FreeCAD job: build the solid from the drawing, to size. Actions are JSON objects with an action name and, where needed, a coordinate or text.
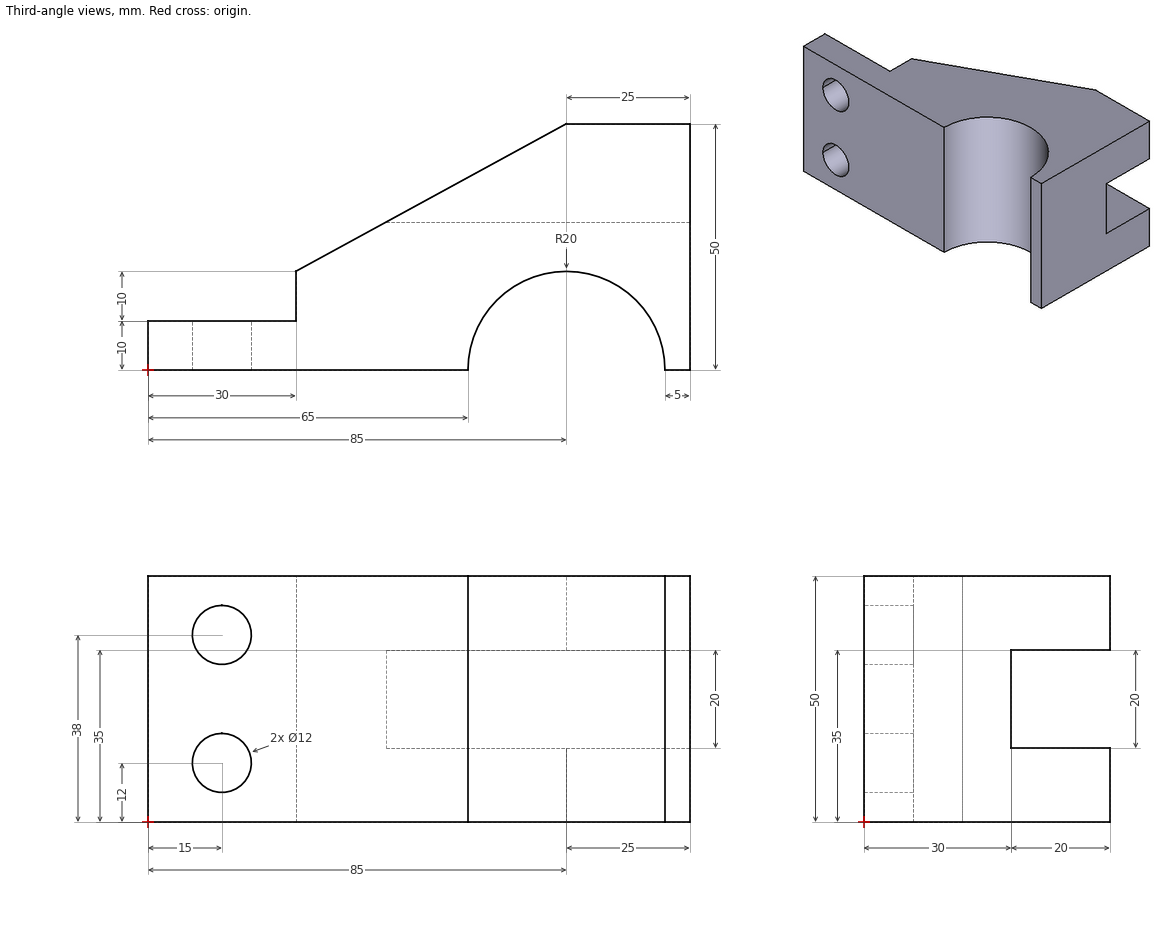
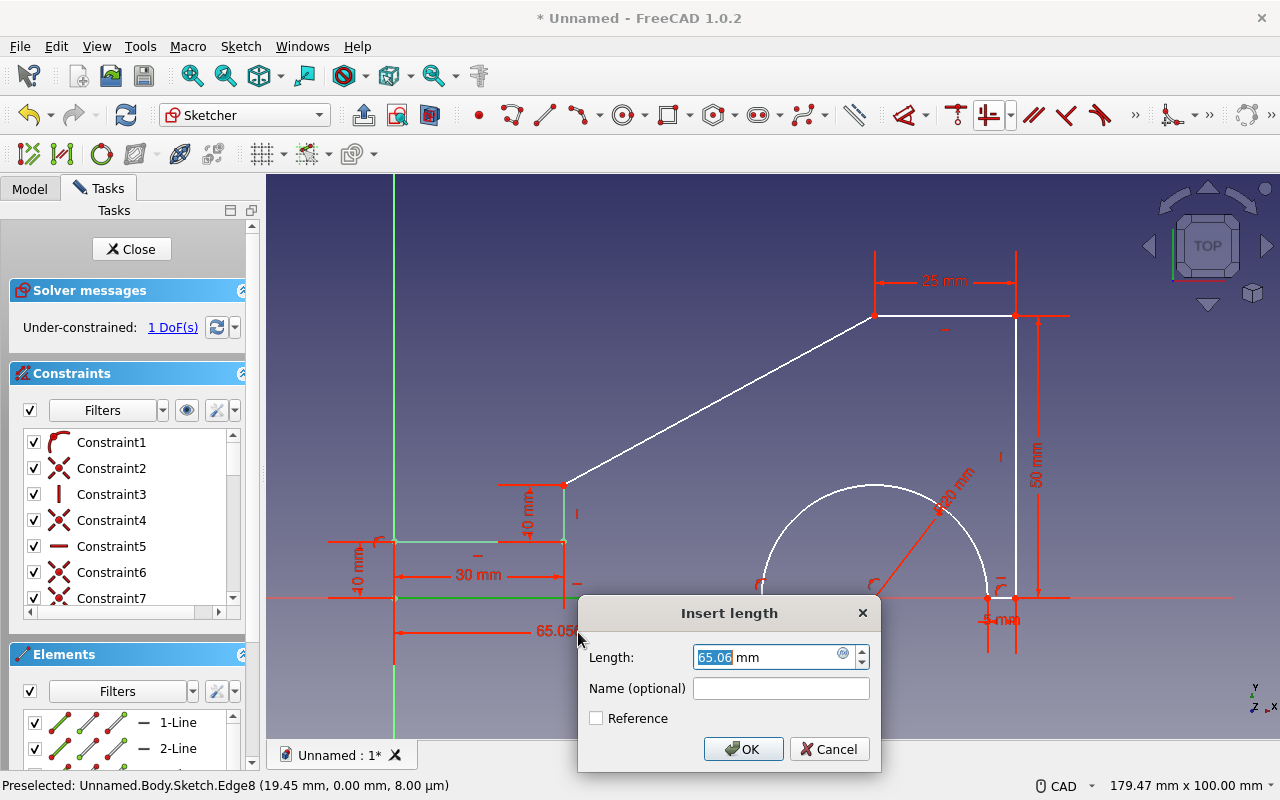
{"action": "type", "text": "65"}
{"action": "key", "text": "Return"}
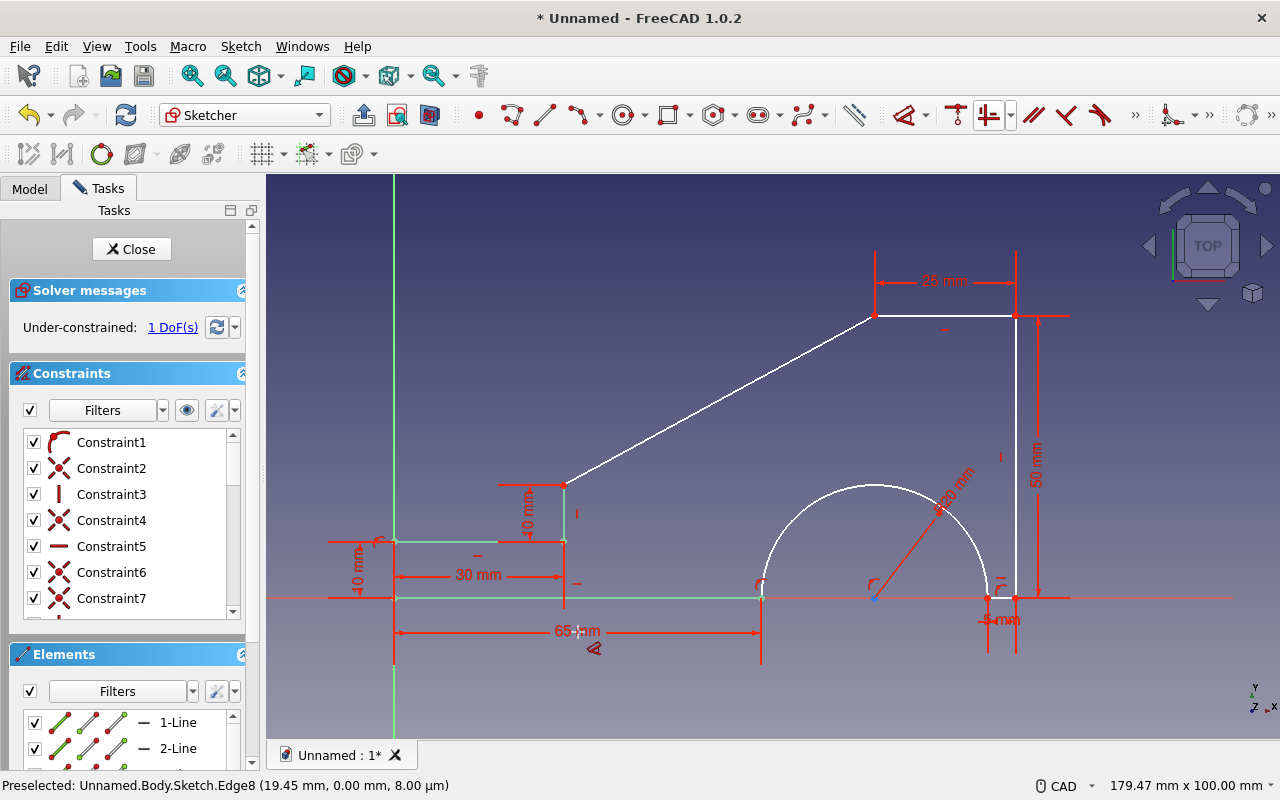
{"action": "left_click", "coordinate": [875, 316]}
{"action": "left_click", "coordinate": [745, 632]}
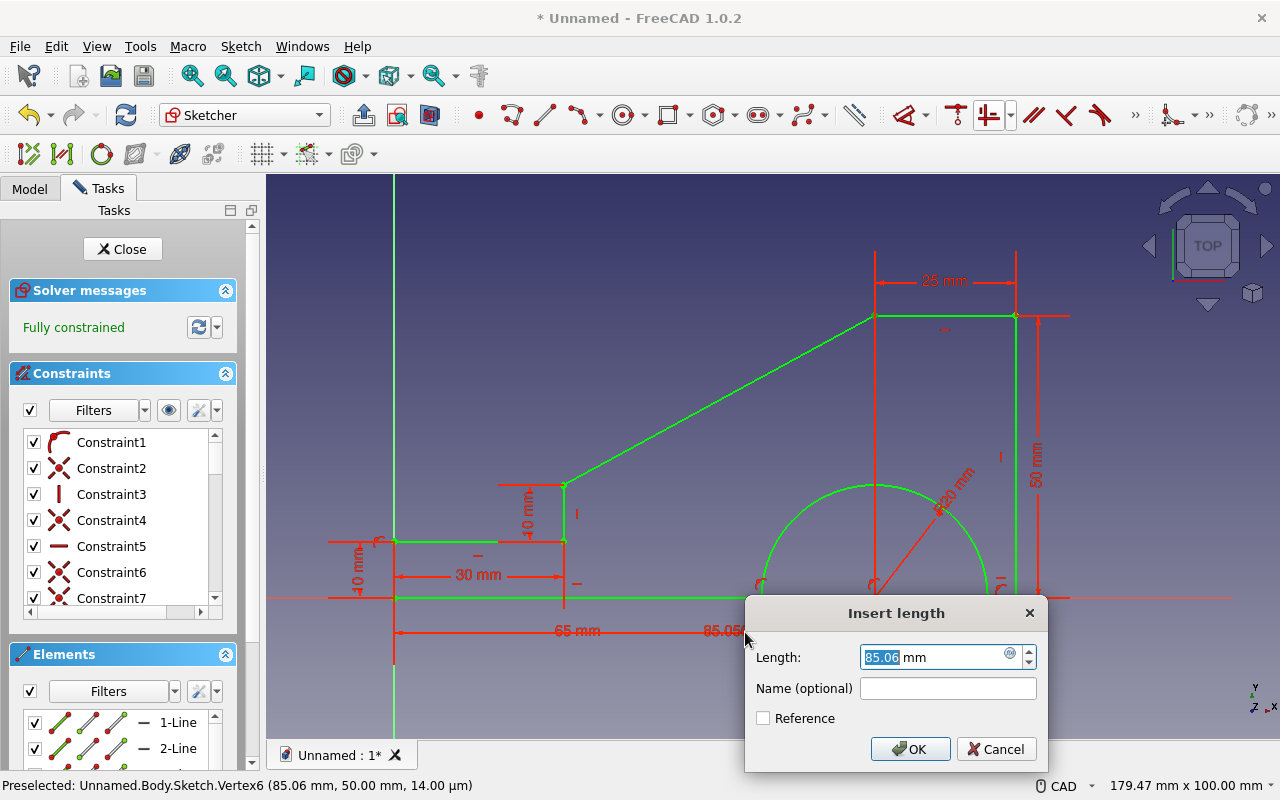
{"action": "type", "text": "85"}
{"action": "key", "text": "Return"}
{"action": "key", "text": "Escape"}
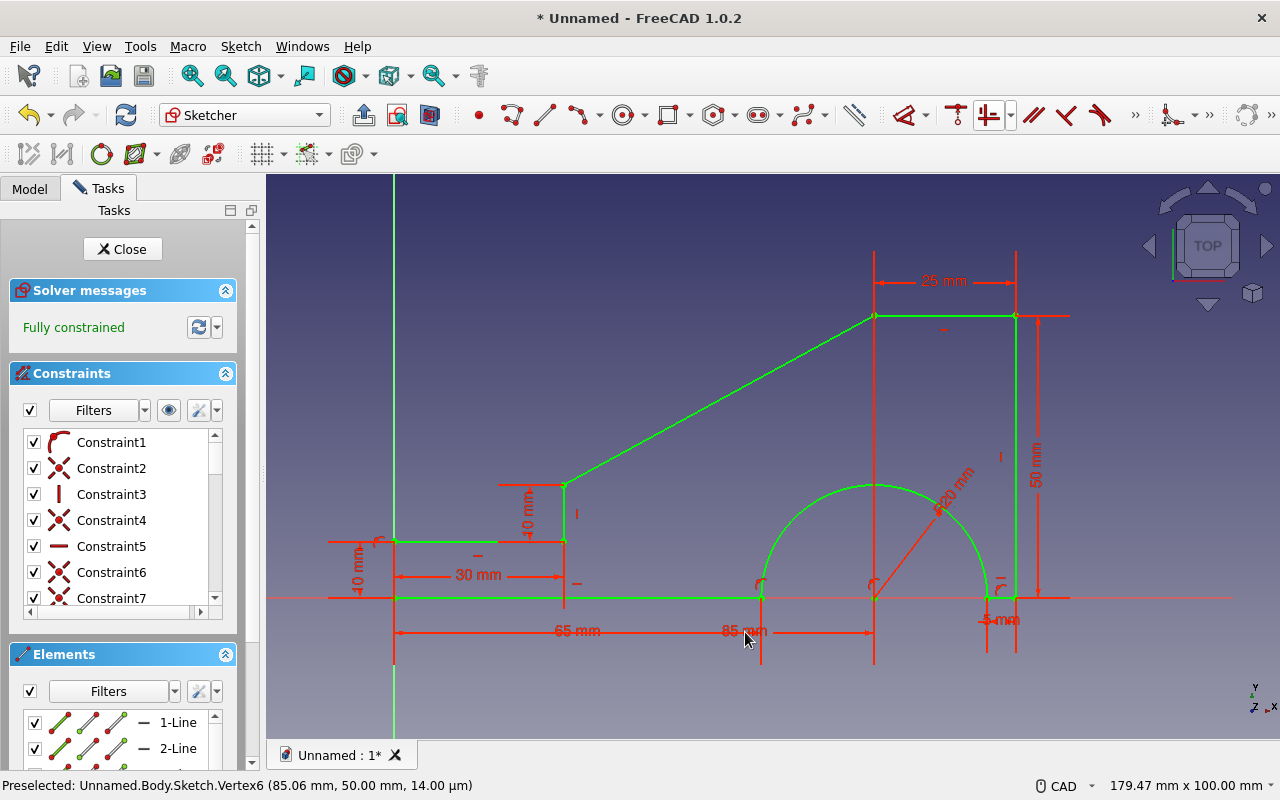
{"action": "left_click", "coordinate": [123, 249]}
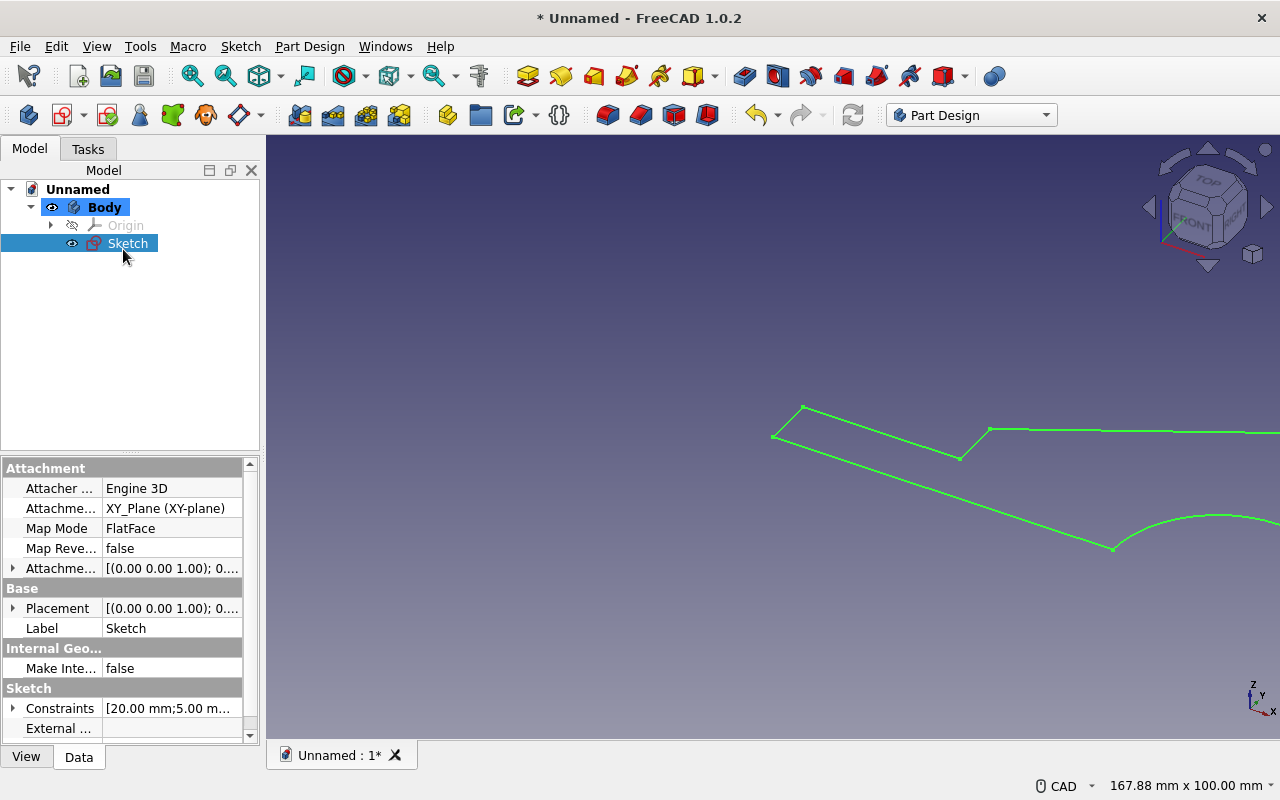
{"action": "left_click", "coordinate": [528, 76]}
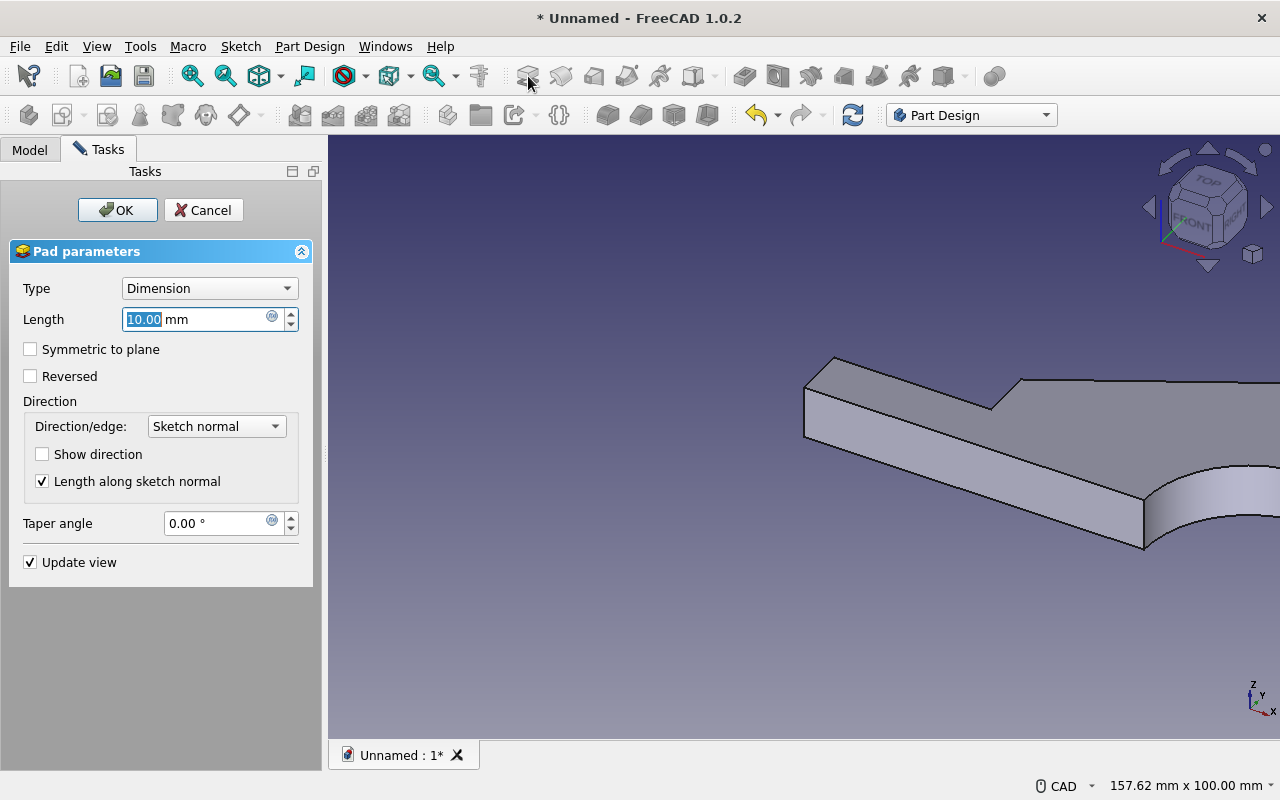
{"action": "type", "text": "50"}
{"action": "key", "text": "Tab"}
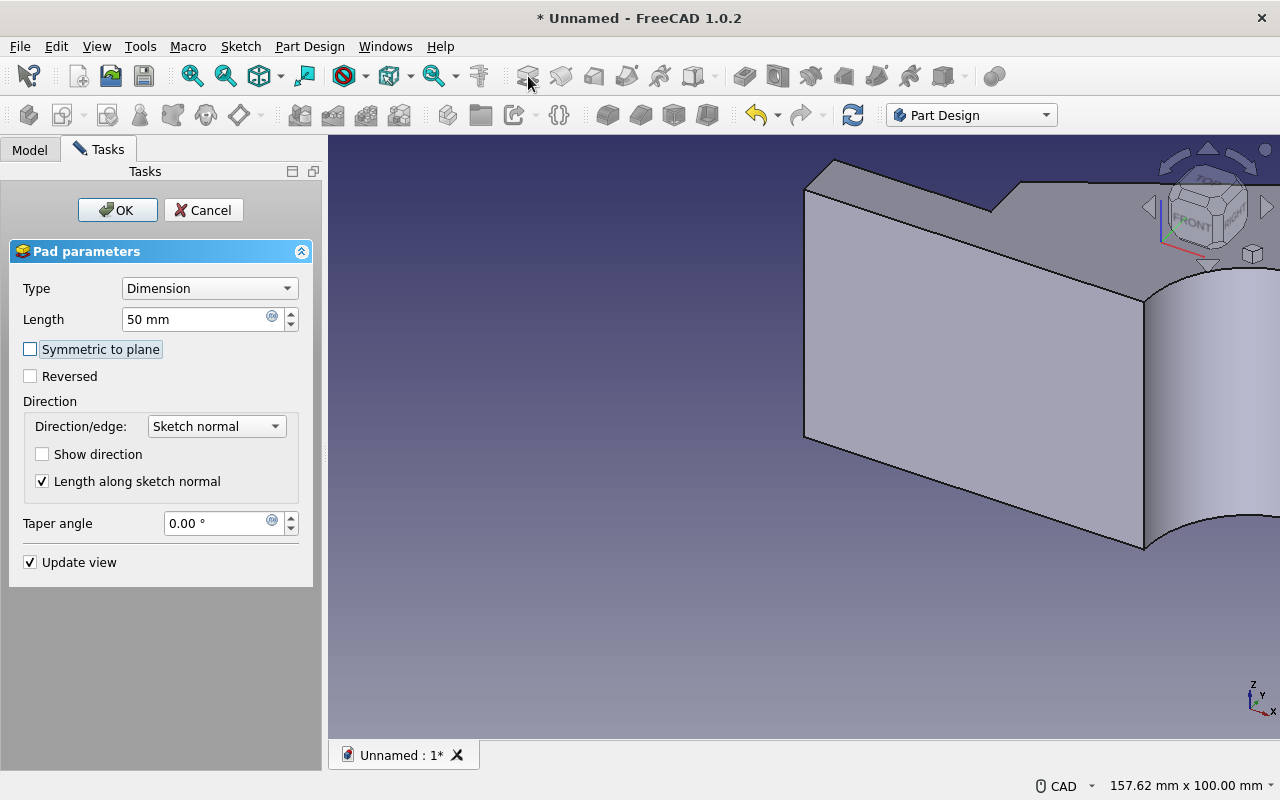
{"action": "left_click", "coordinate": [118, 210]}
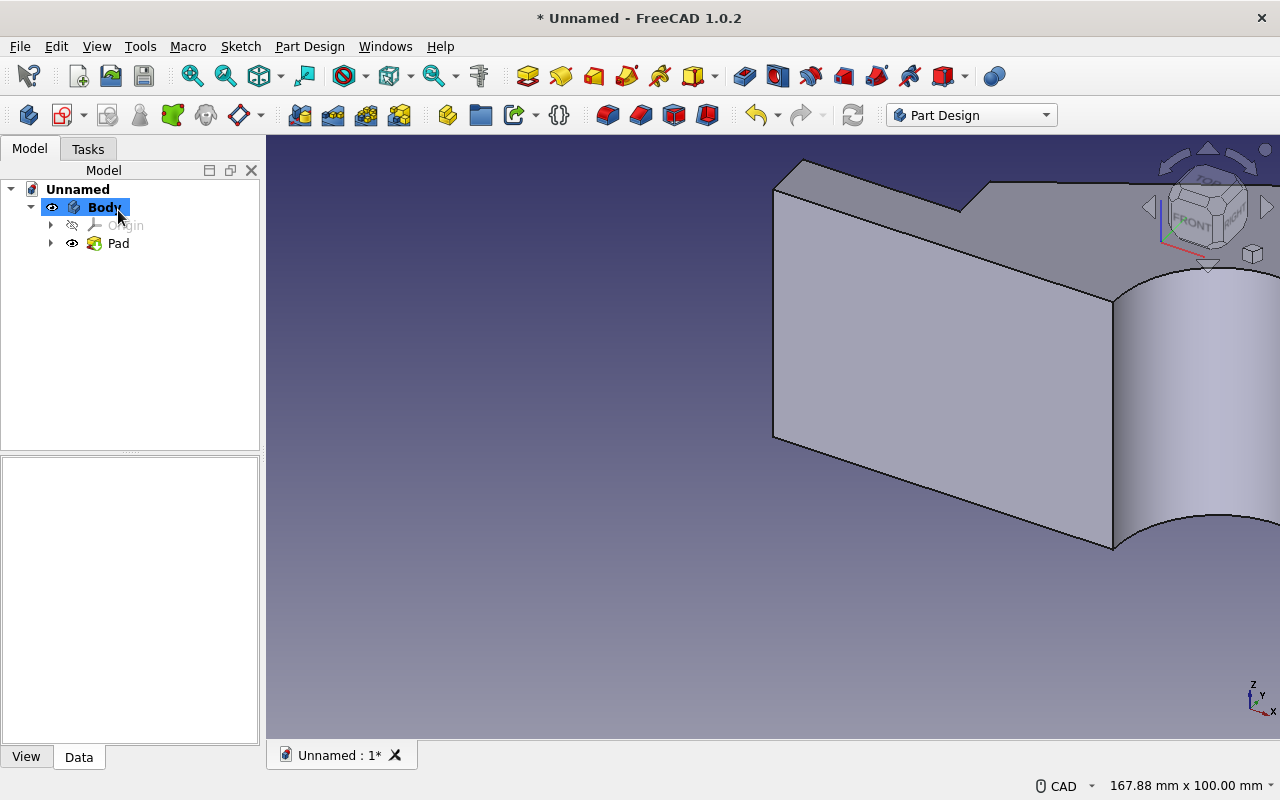
{"action": "left_click", "coordinate": [193, 76]}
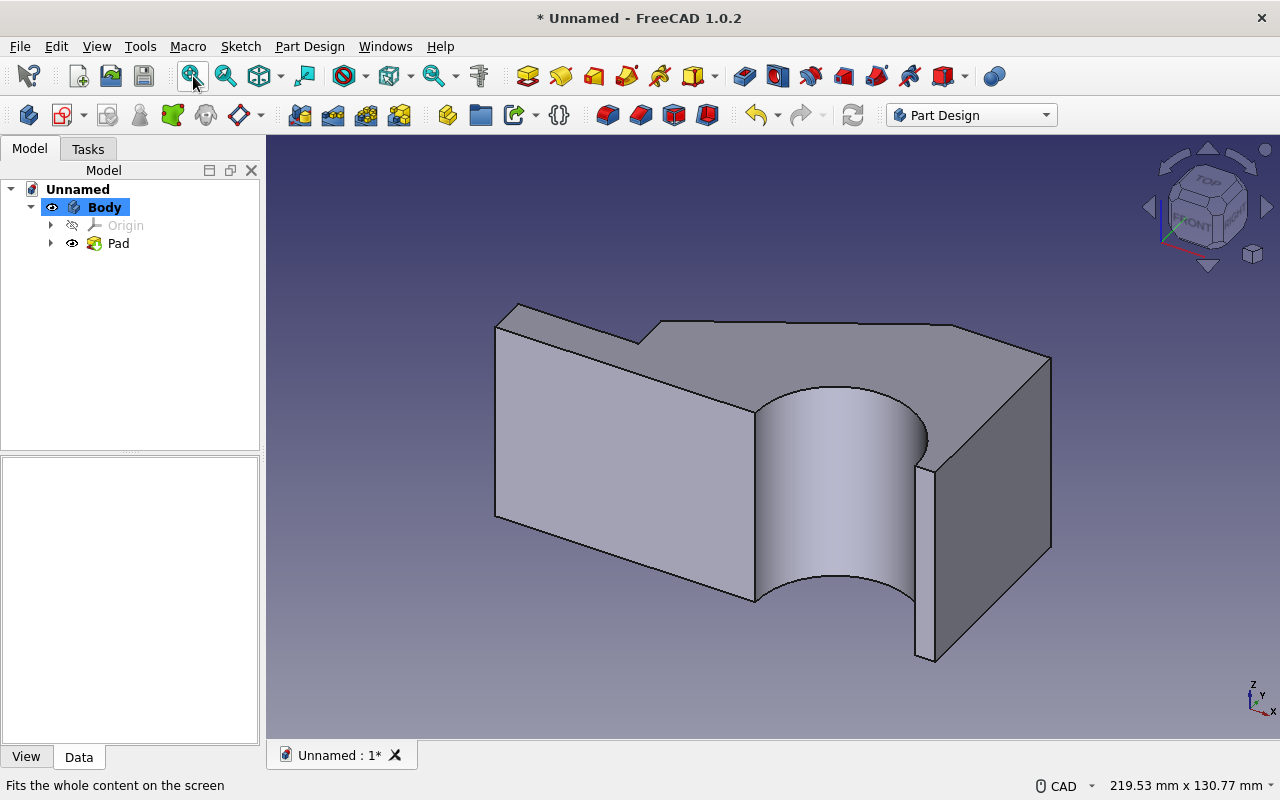
{"action": "key", "text": "4"}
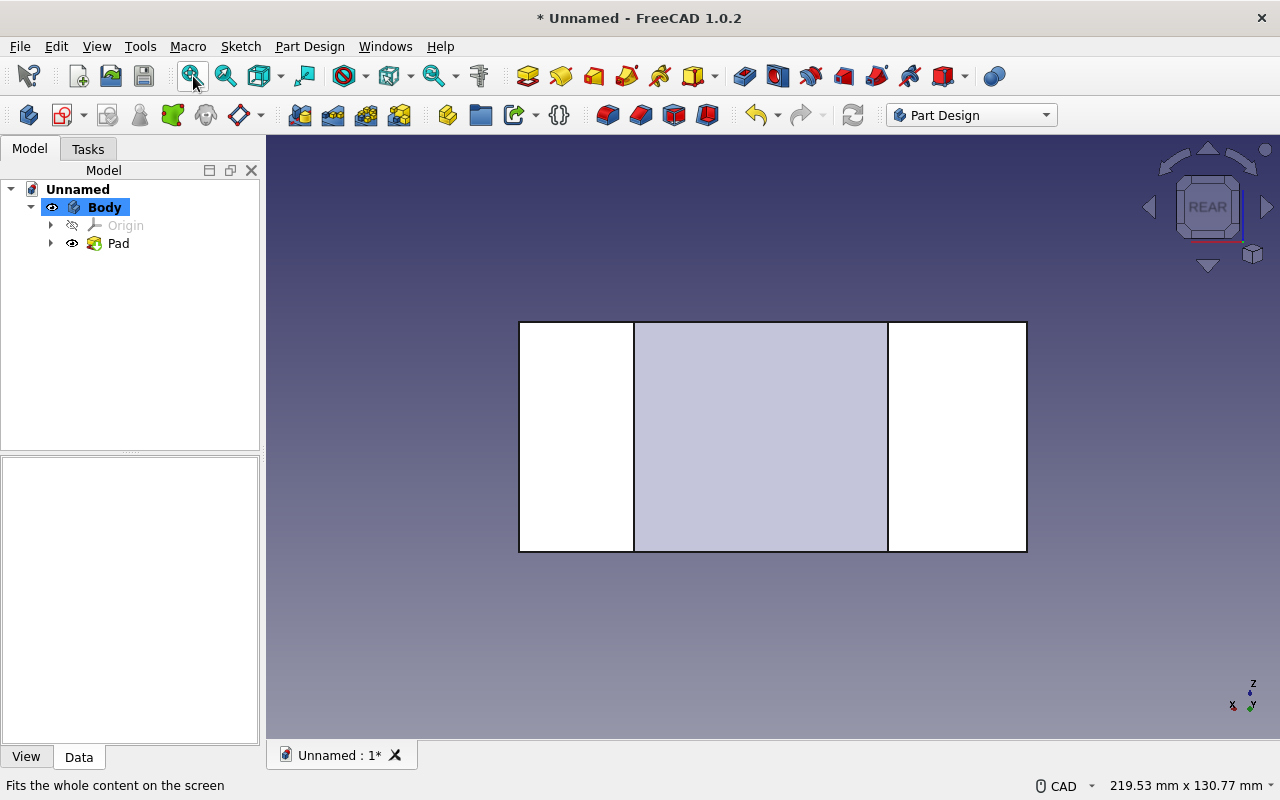
{"action": "left_click", "coordinate": [577, 403]}